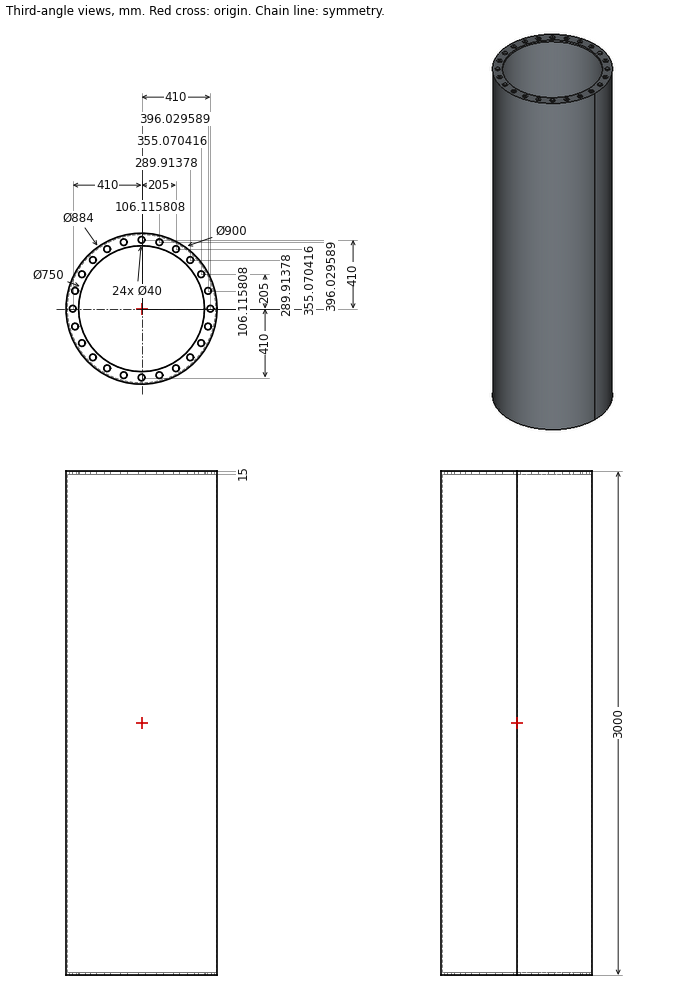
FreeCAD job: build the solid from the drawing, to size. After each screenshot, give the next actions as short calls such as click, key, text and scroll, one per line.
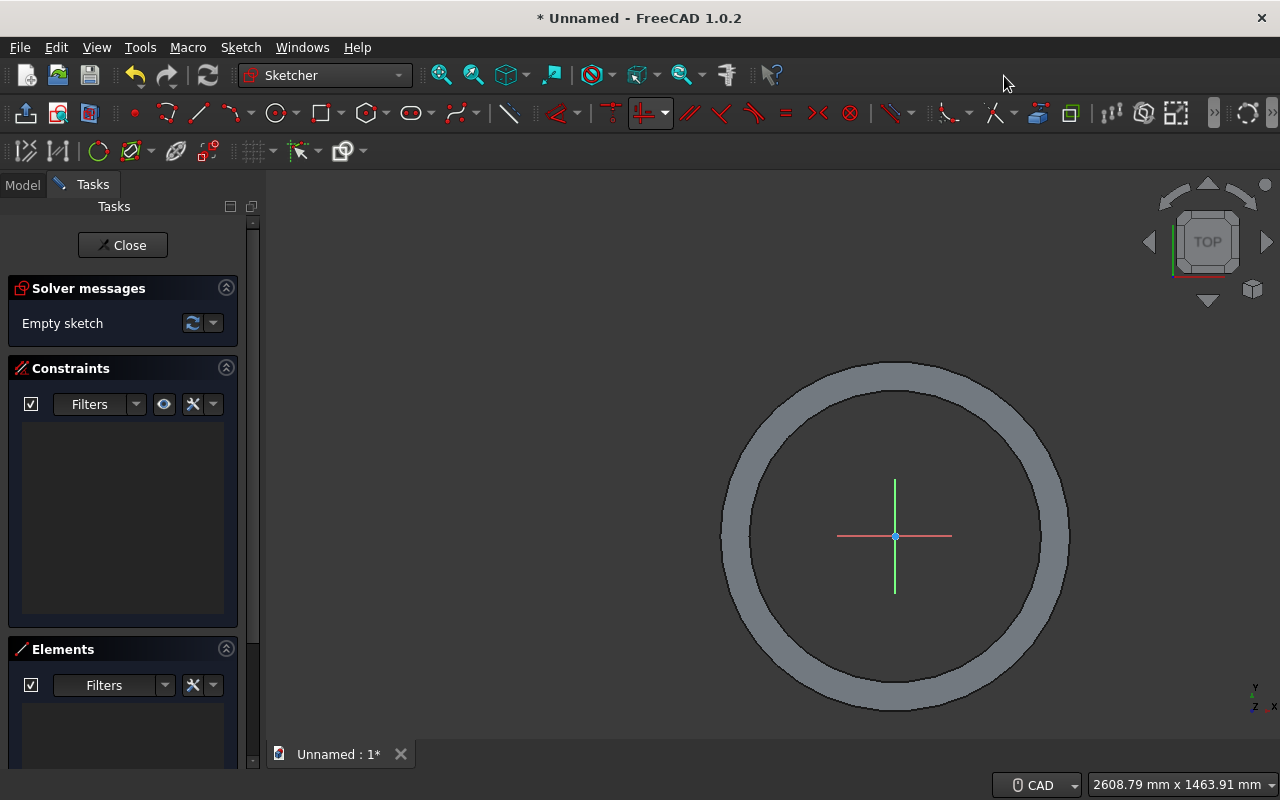
scroll(294, 198, down, 1)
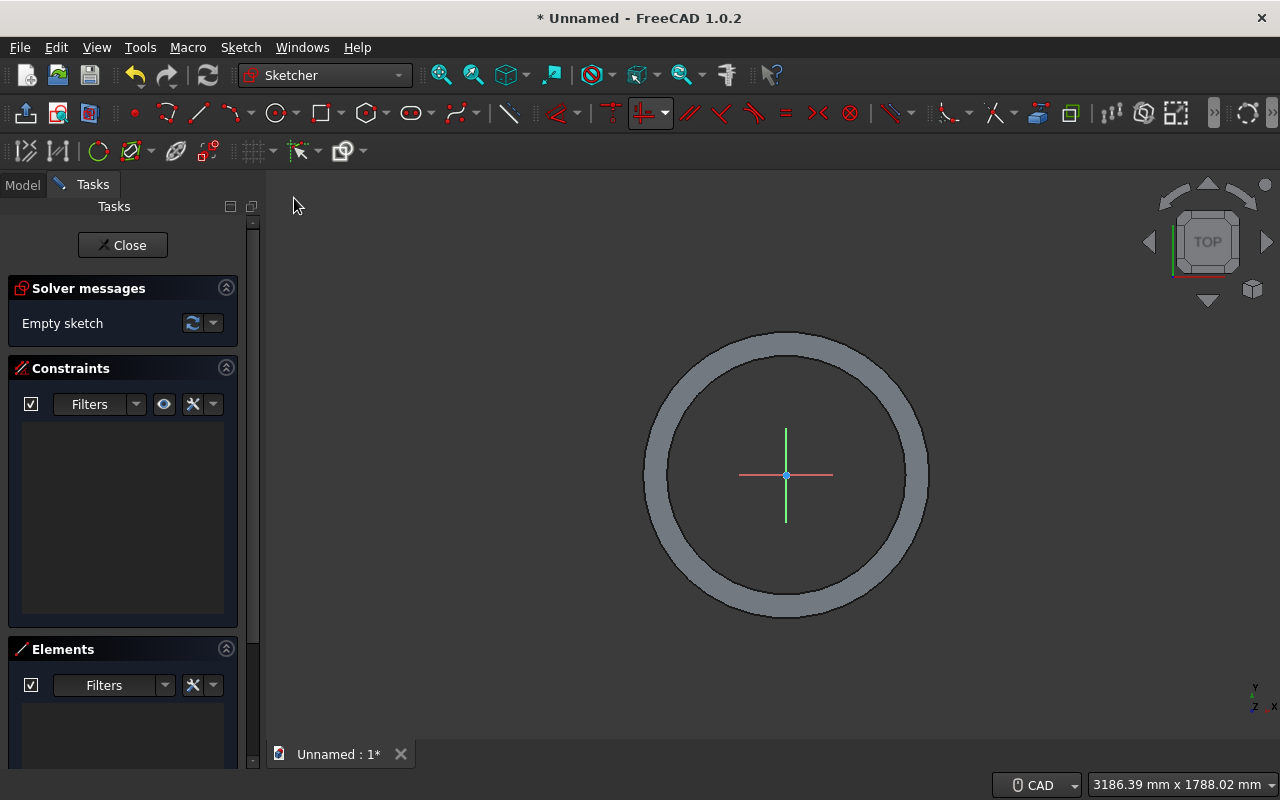
click(276, 114)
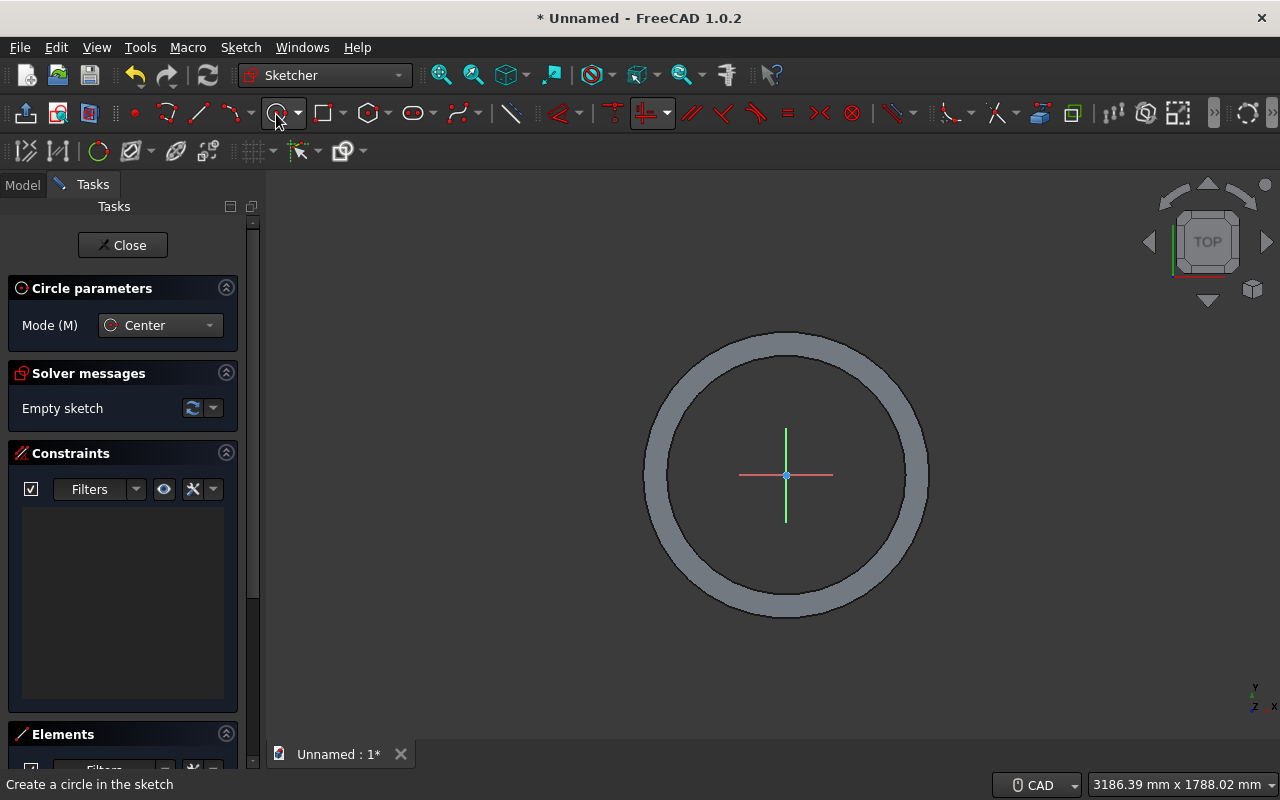
scroll(786, 345, up, 7)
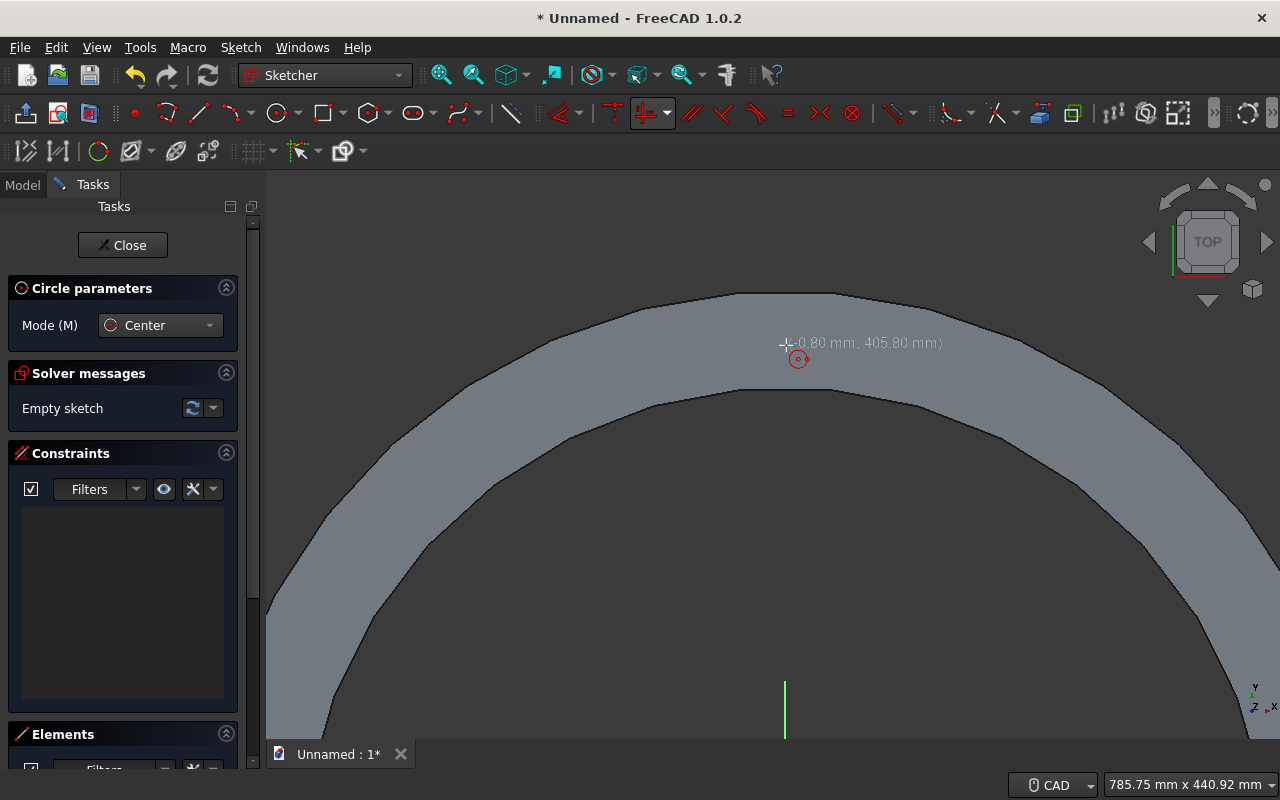
scroll(670, 275, down, 6)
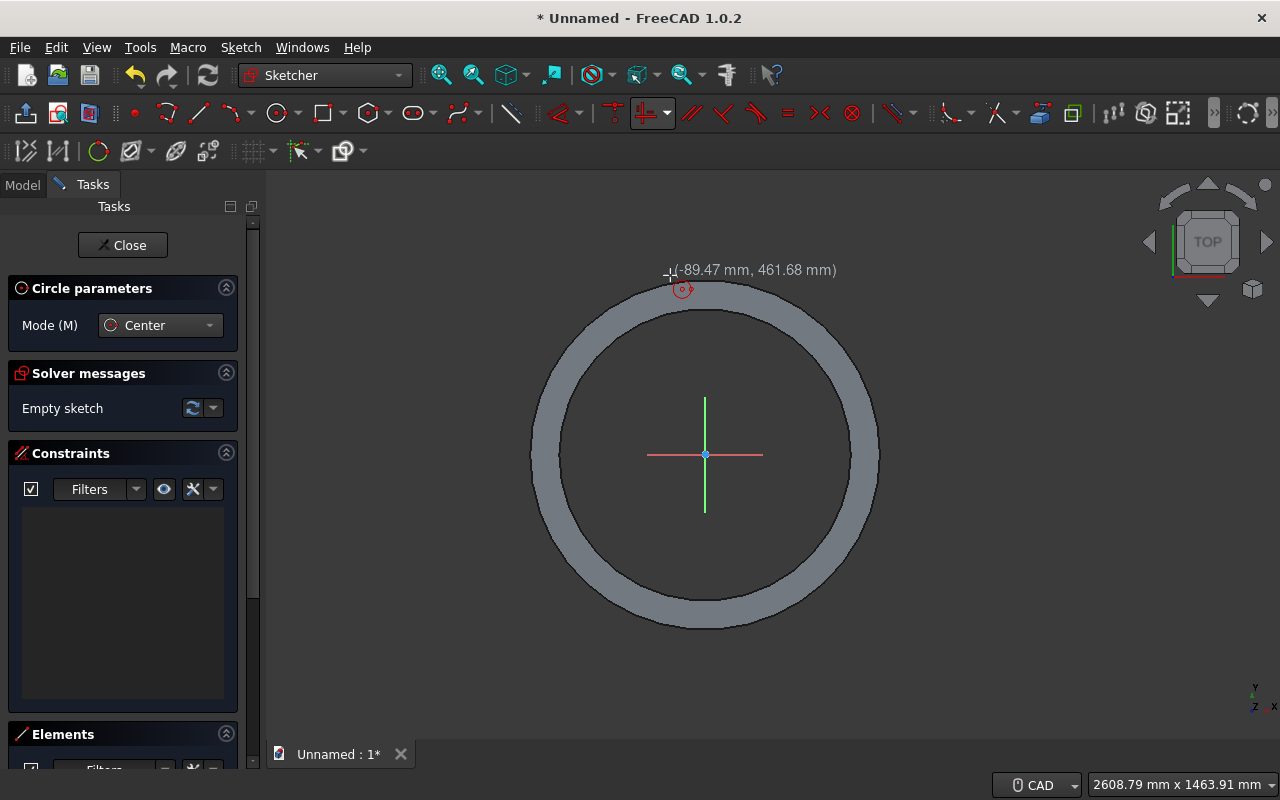
click(705, 296)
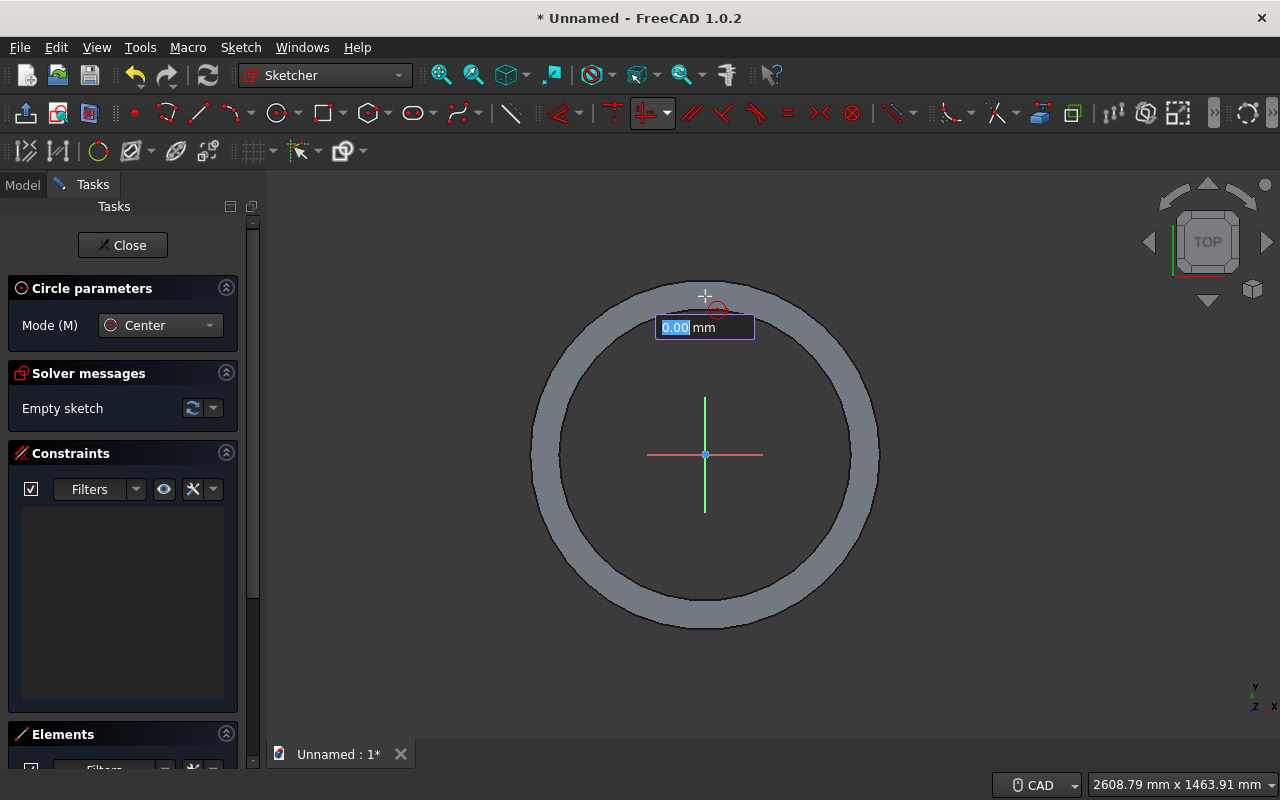
scroll(712, 293, up, 4)
move(712, 292)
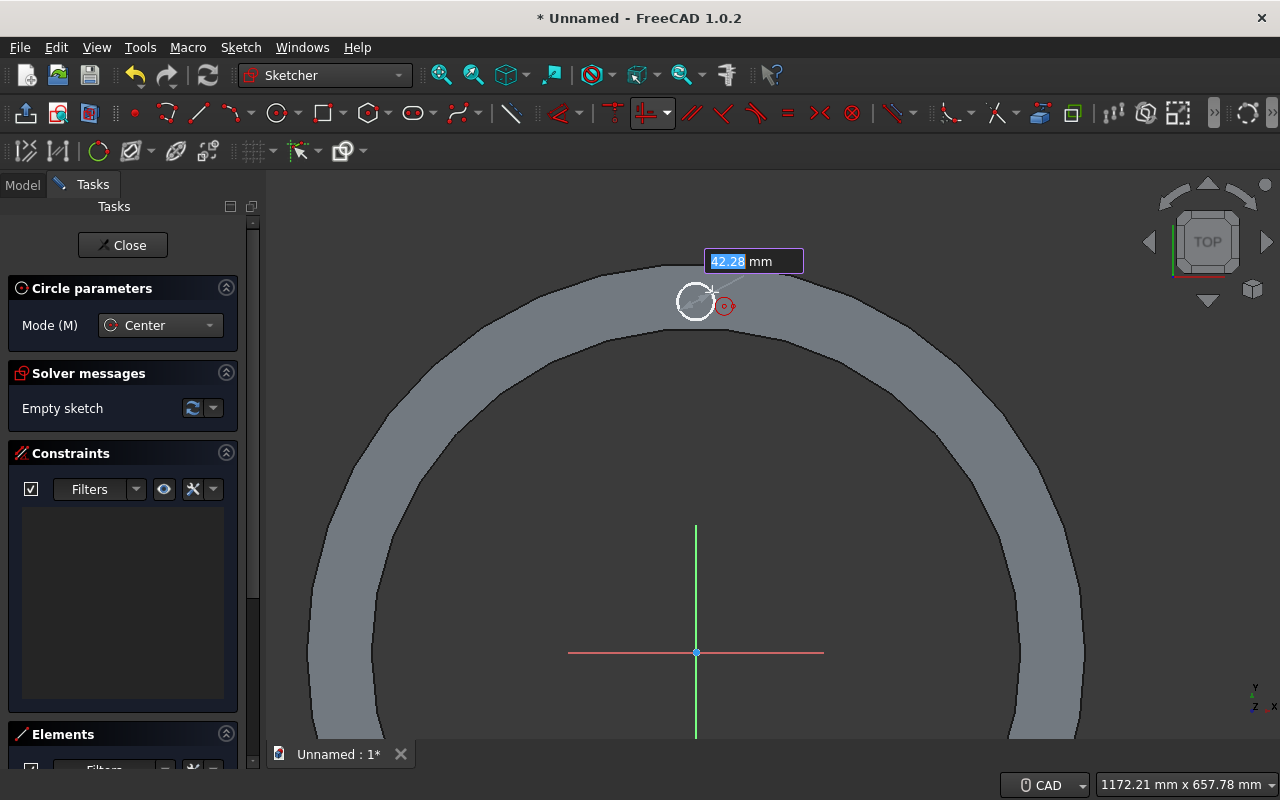
text(40)
key(Return)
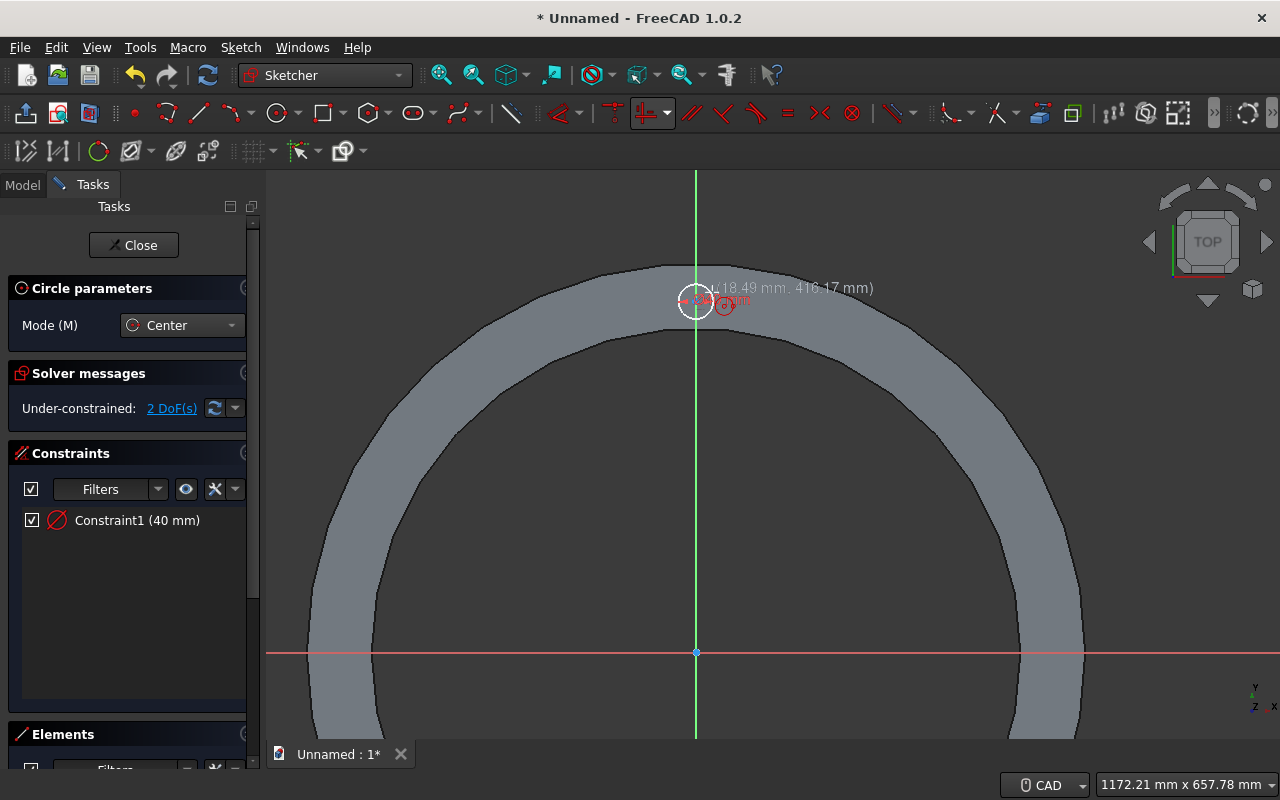
scroll(788, 310, up, 2)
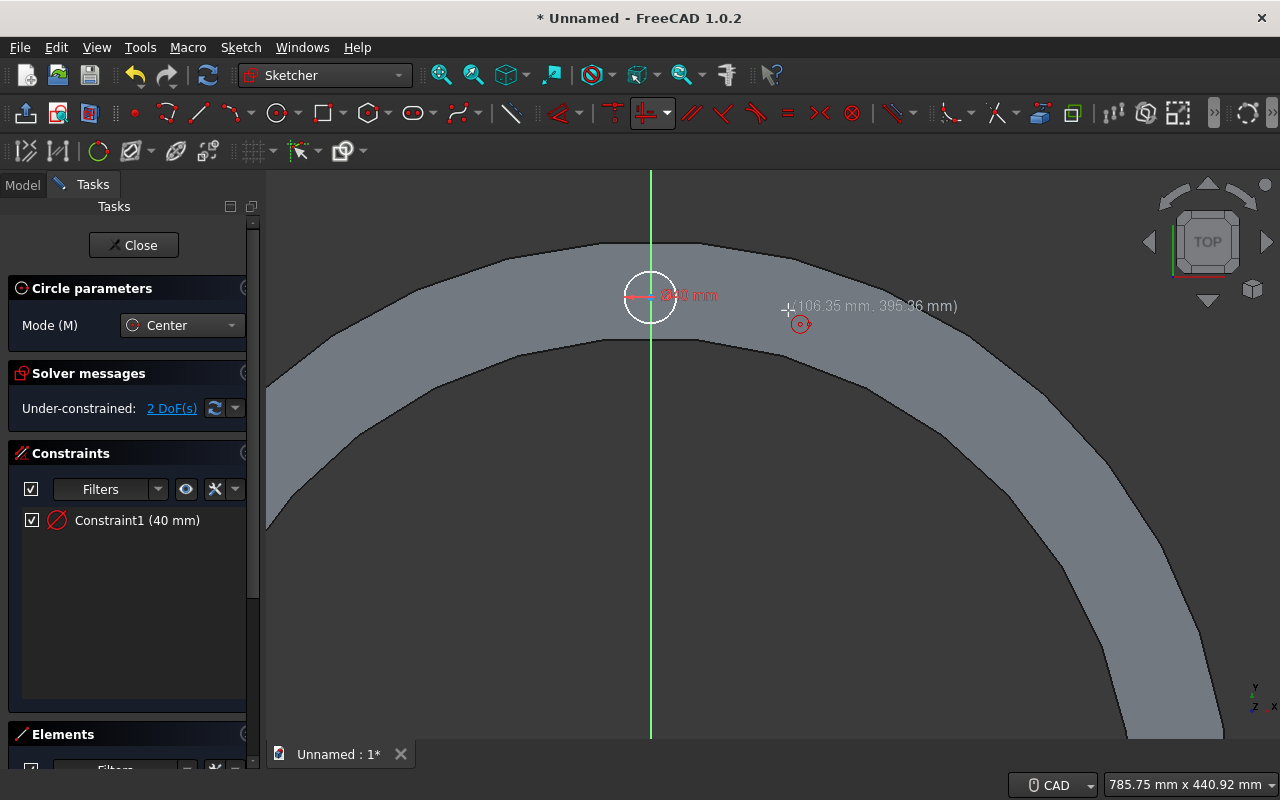
scroll(728, 296, down, 6)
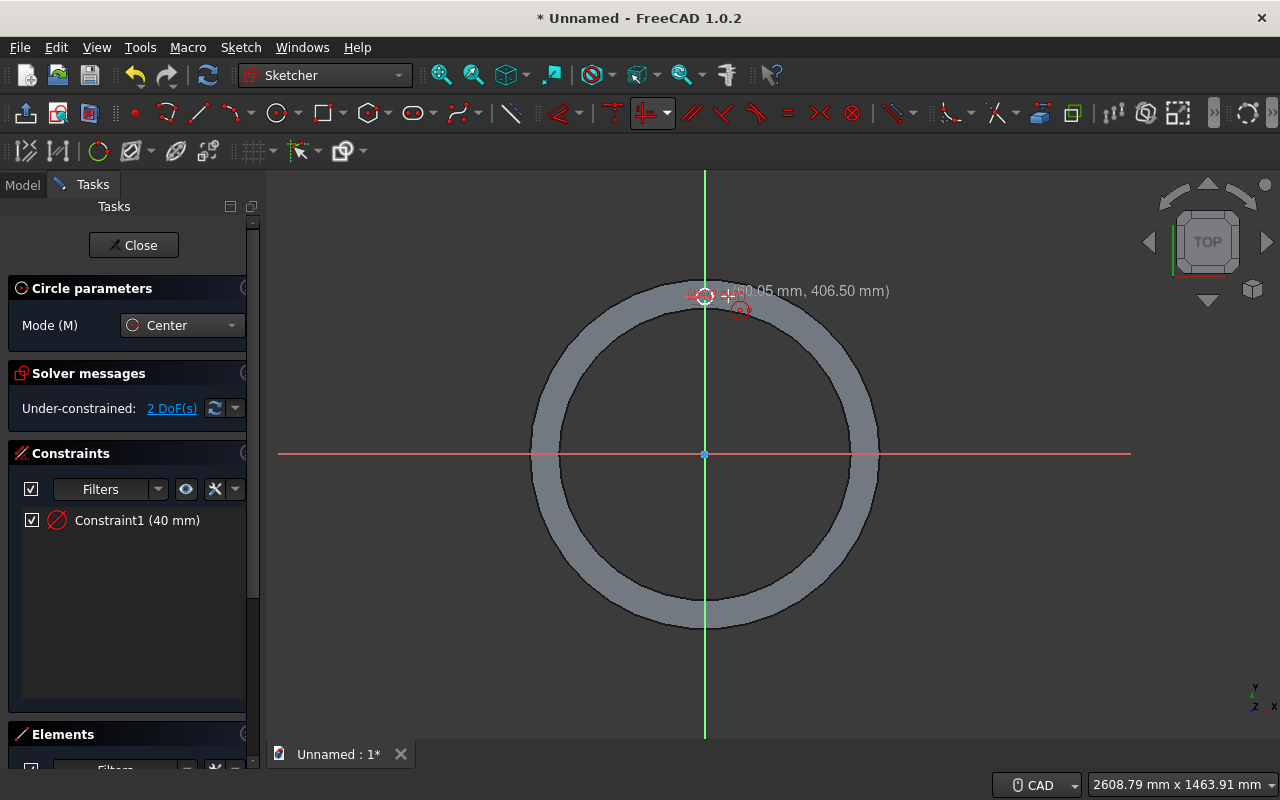
click(746, 301)
move(752, 295)